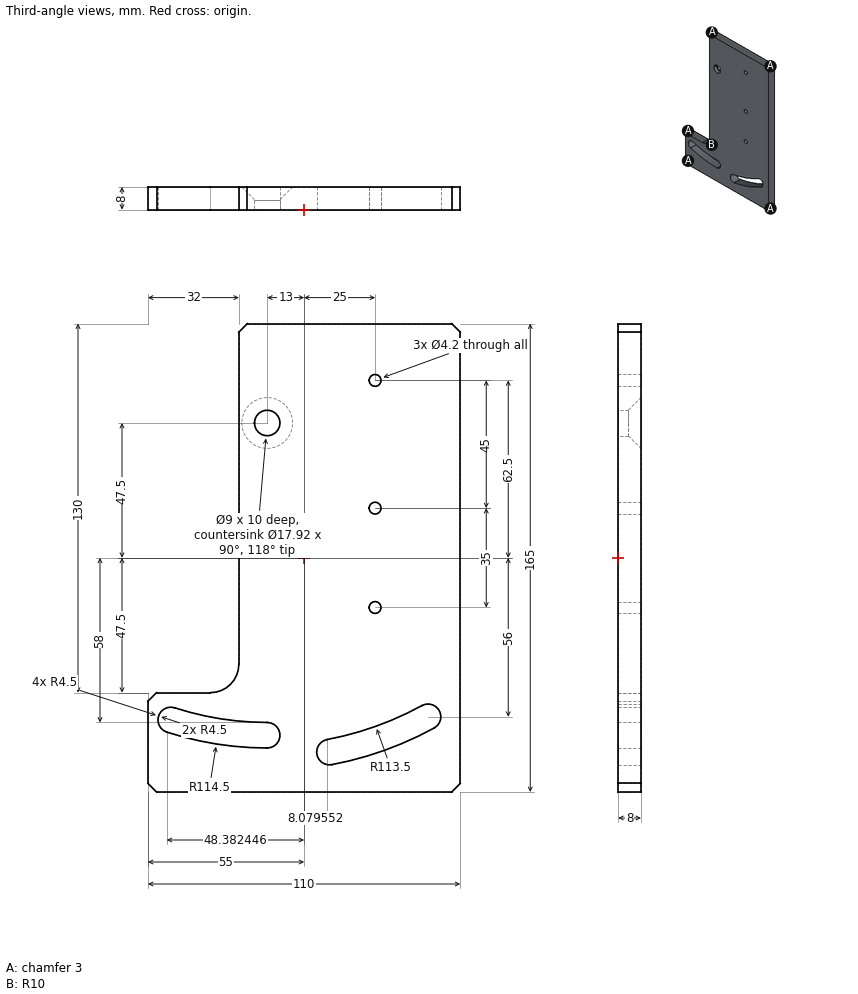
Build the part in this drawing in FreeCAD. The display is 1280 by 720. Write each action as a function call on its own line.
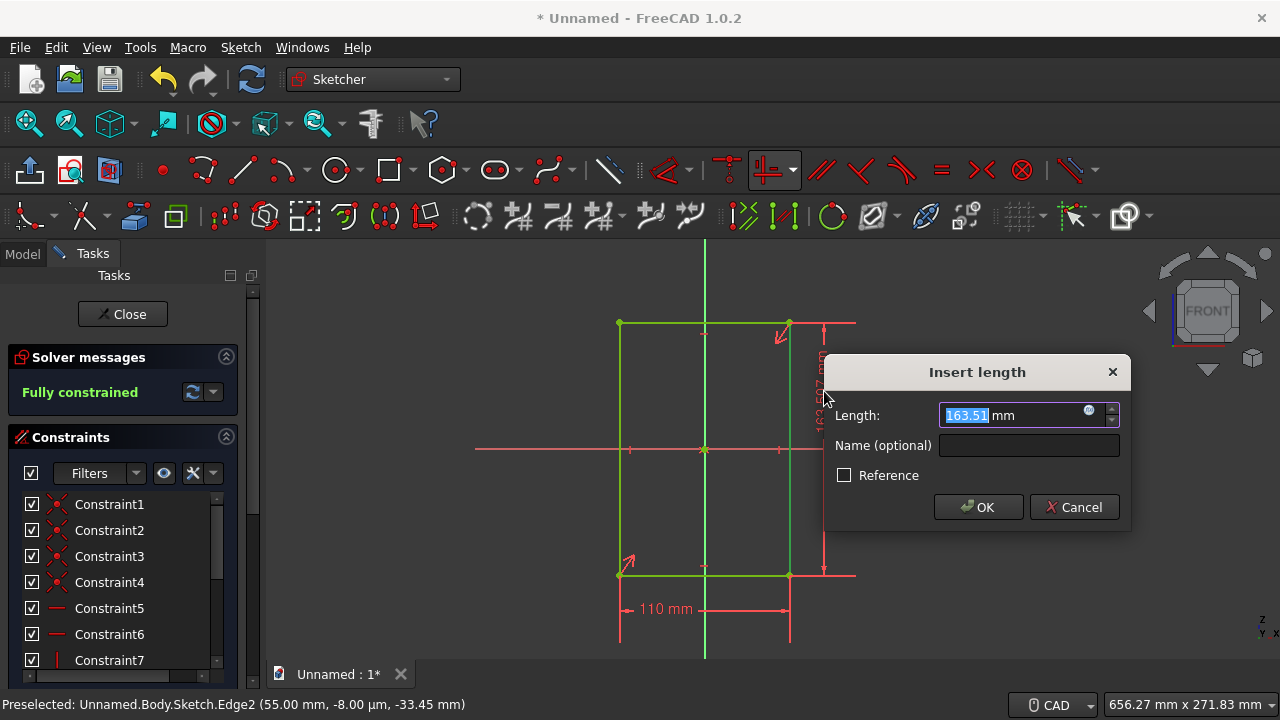
text(165)
key(Return)
key(Escape)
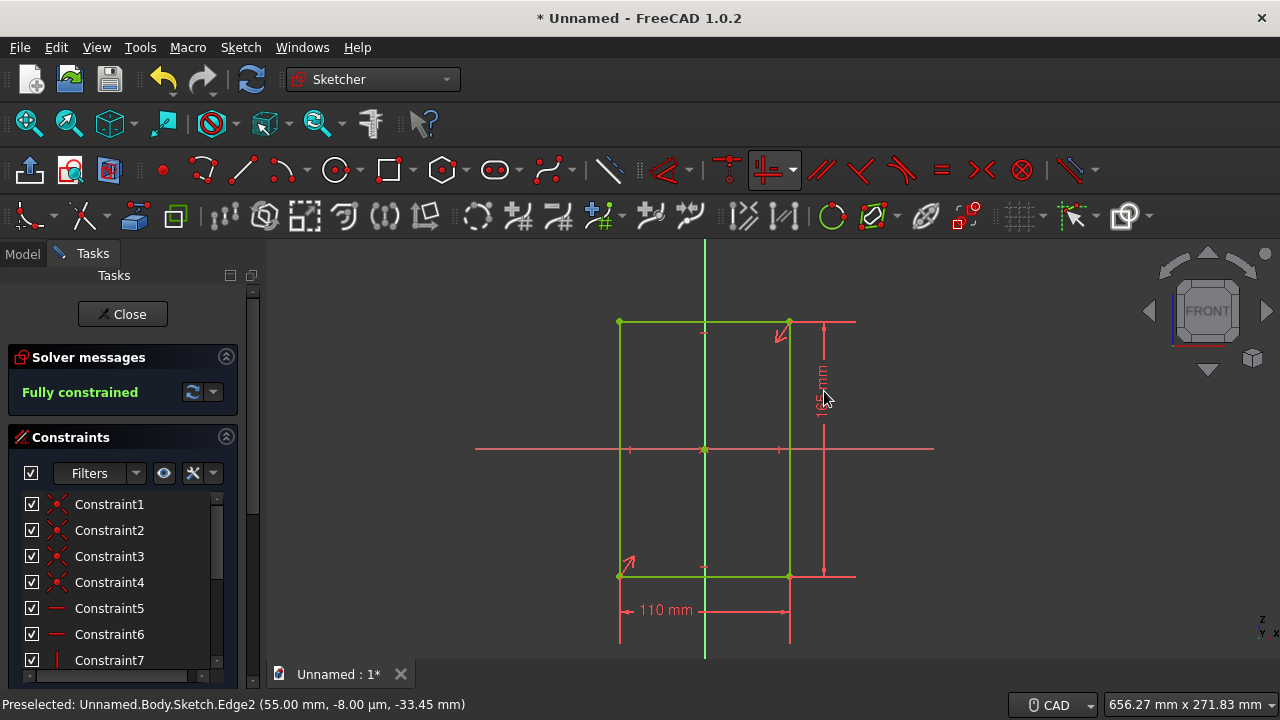
click(123, 314)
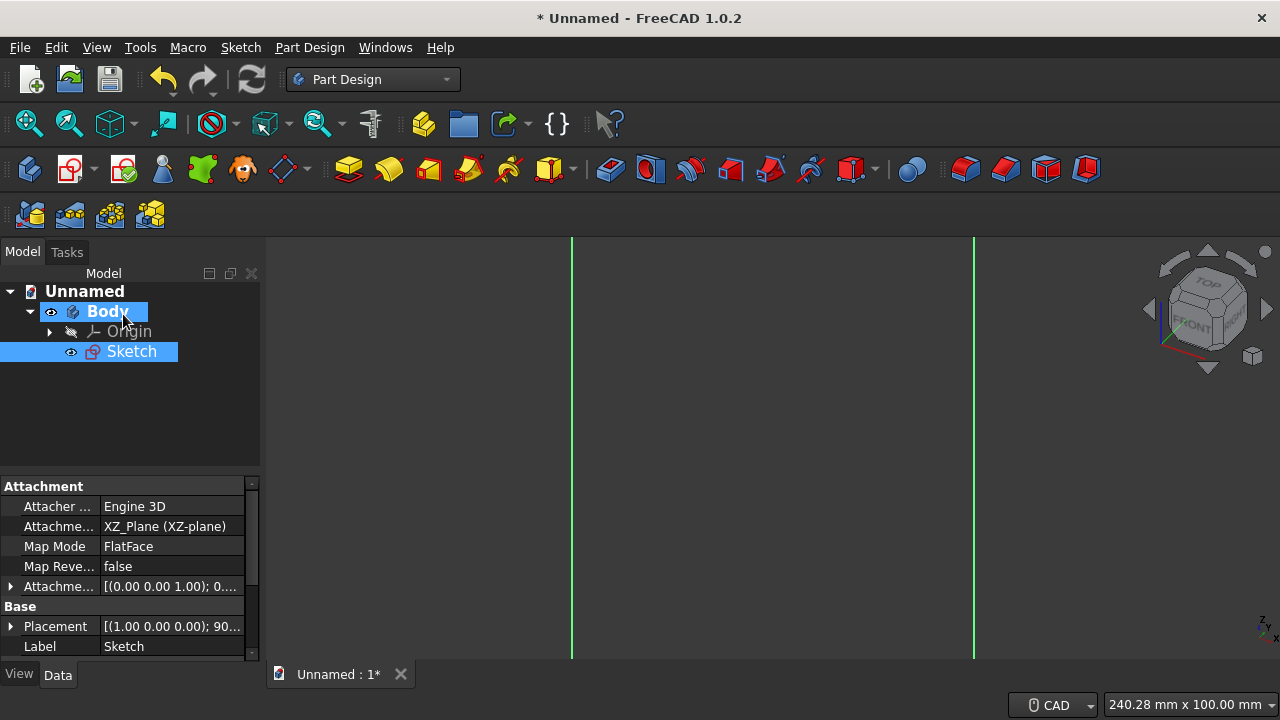
click(350, 170)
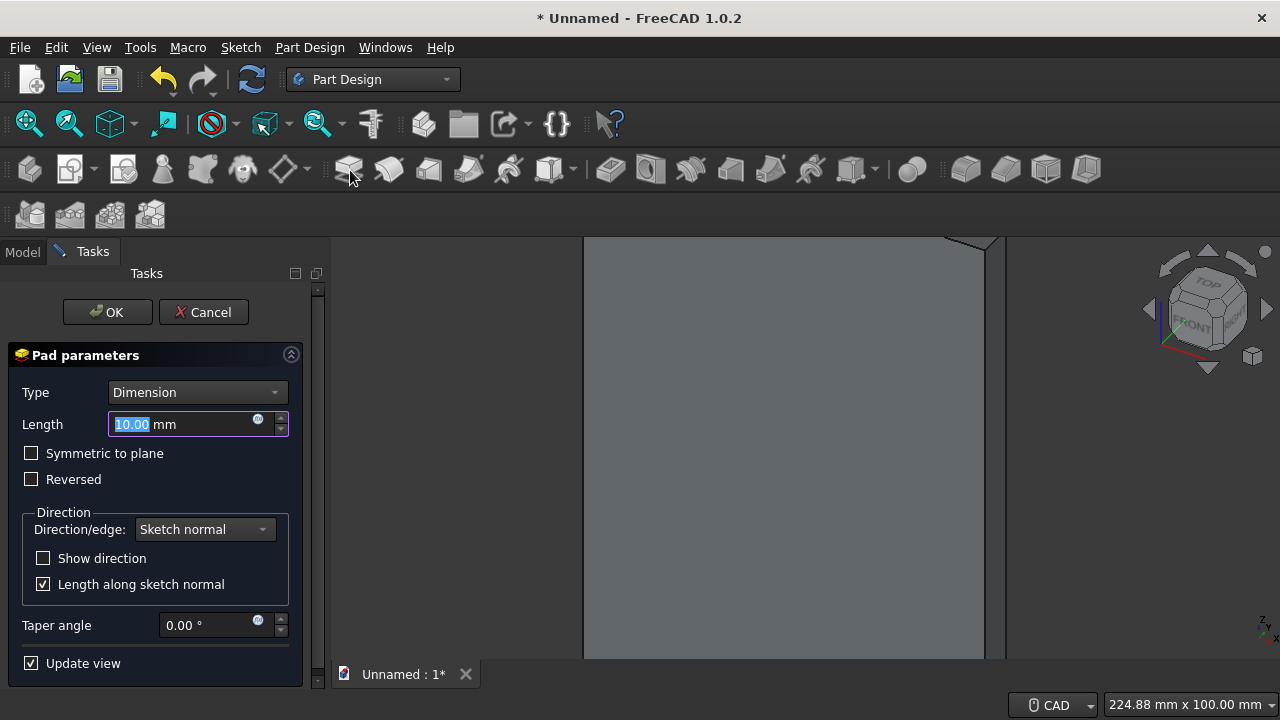
text(8)
key(Tab)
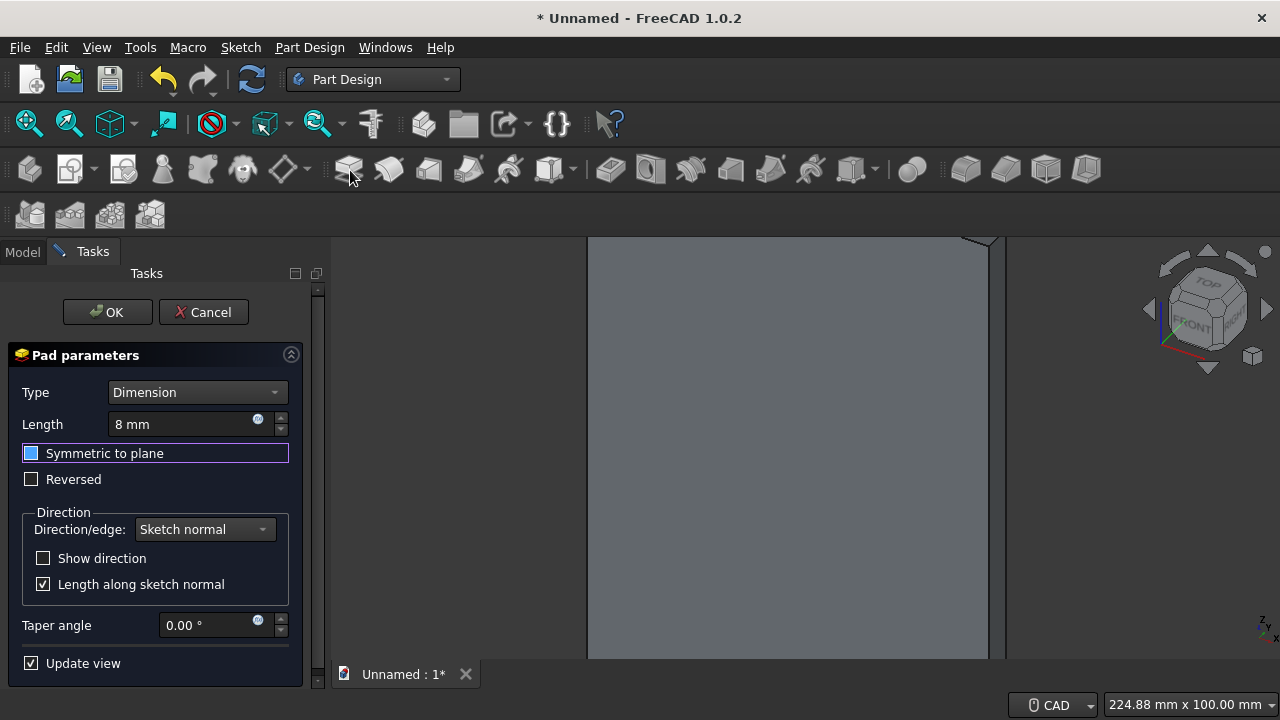
click(30, 479)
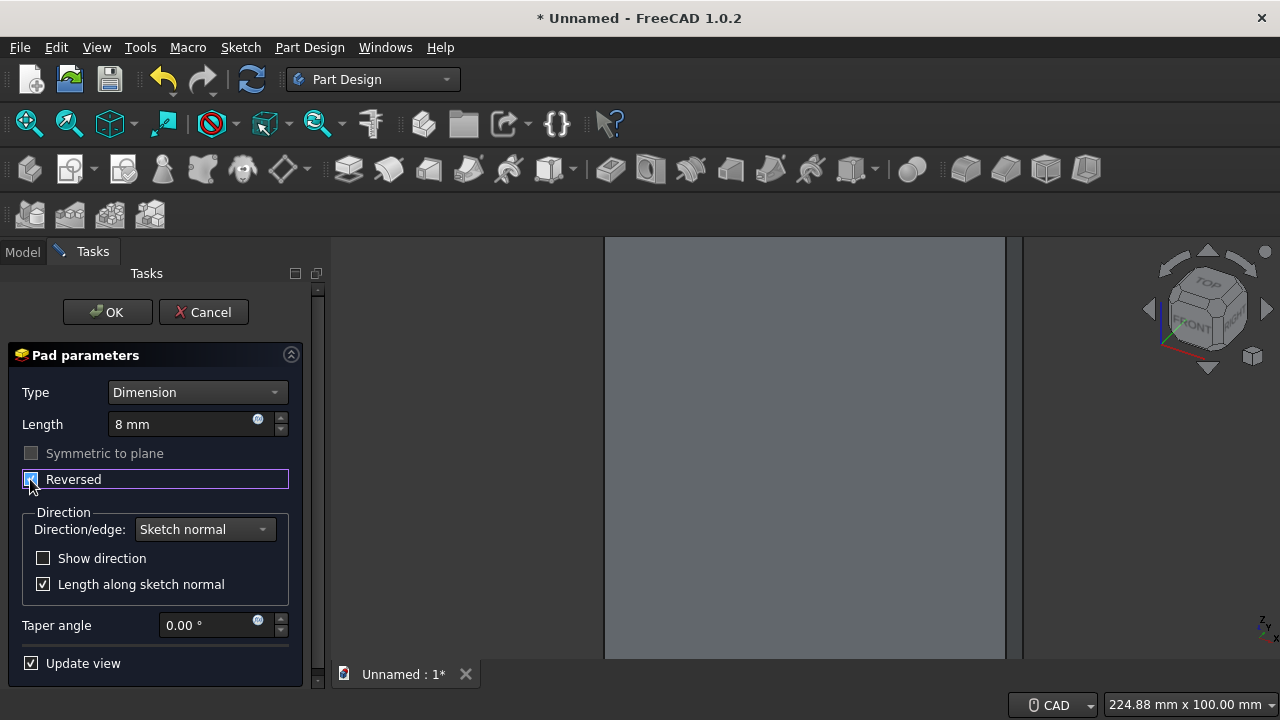
click(108, 312)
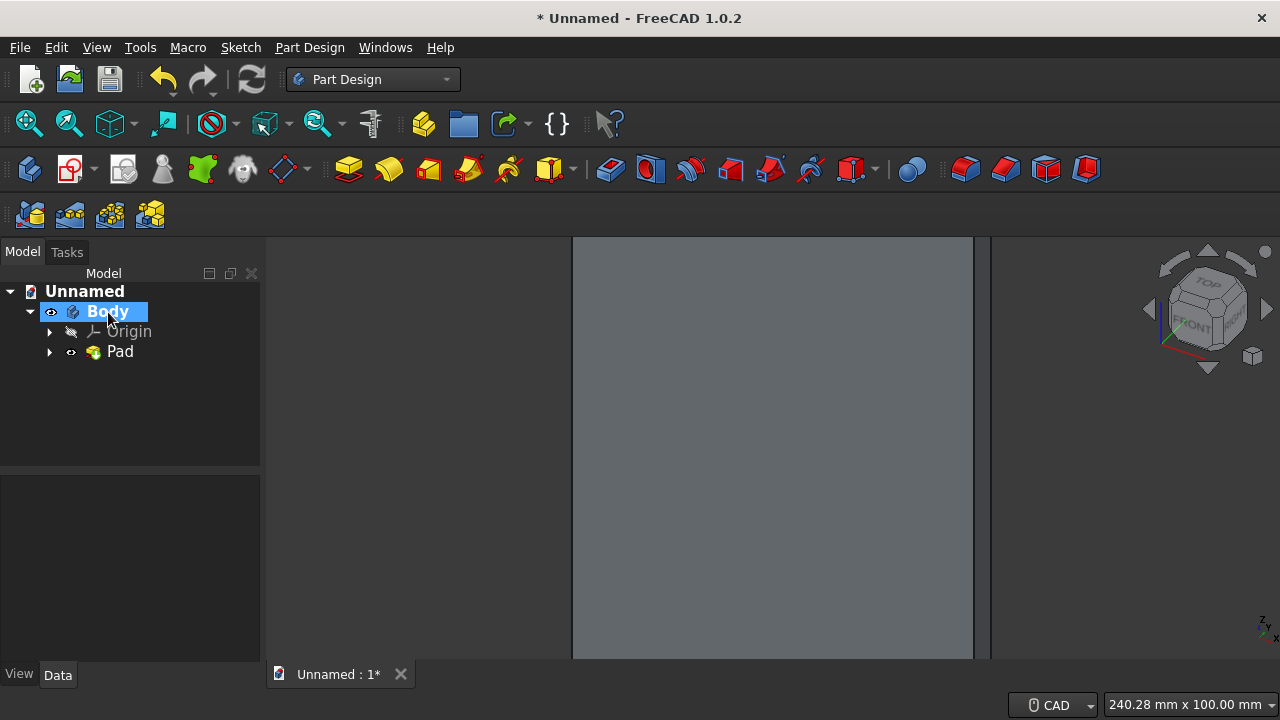
click(30, 124)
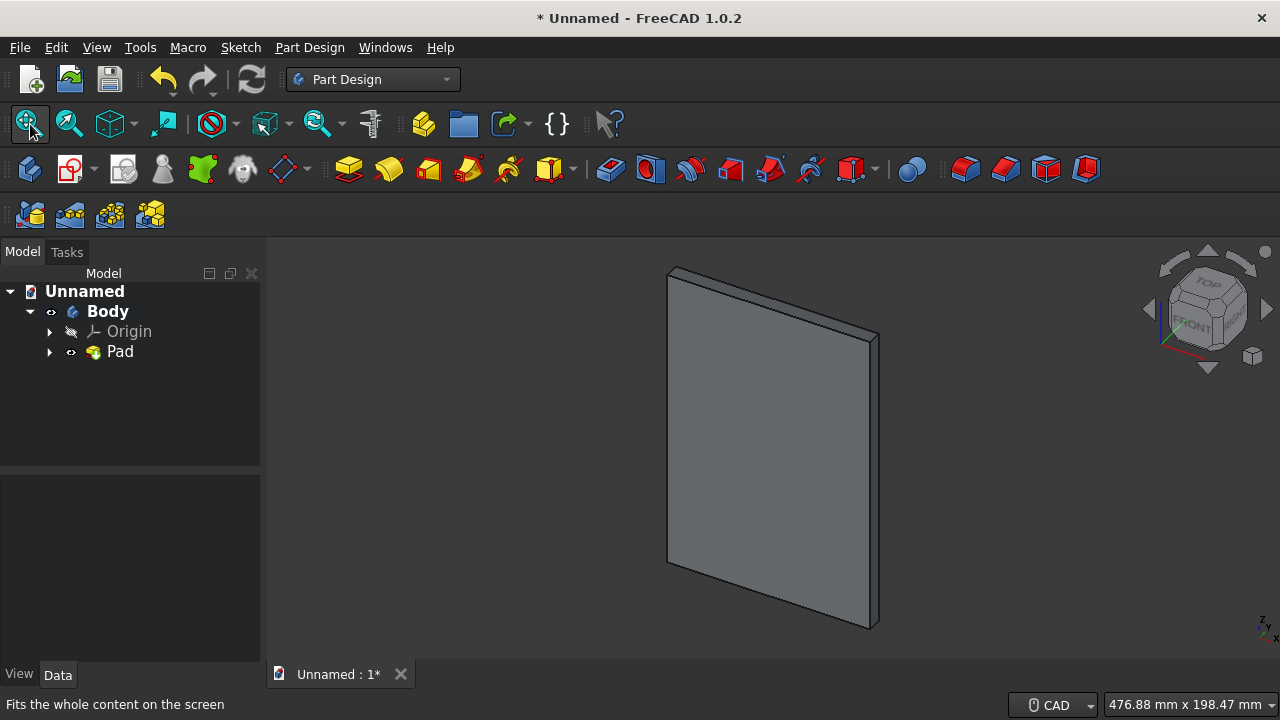
key(4)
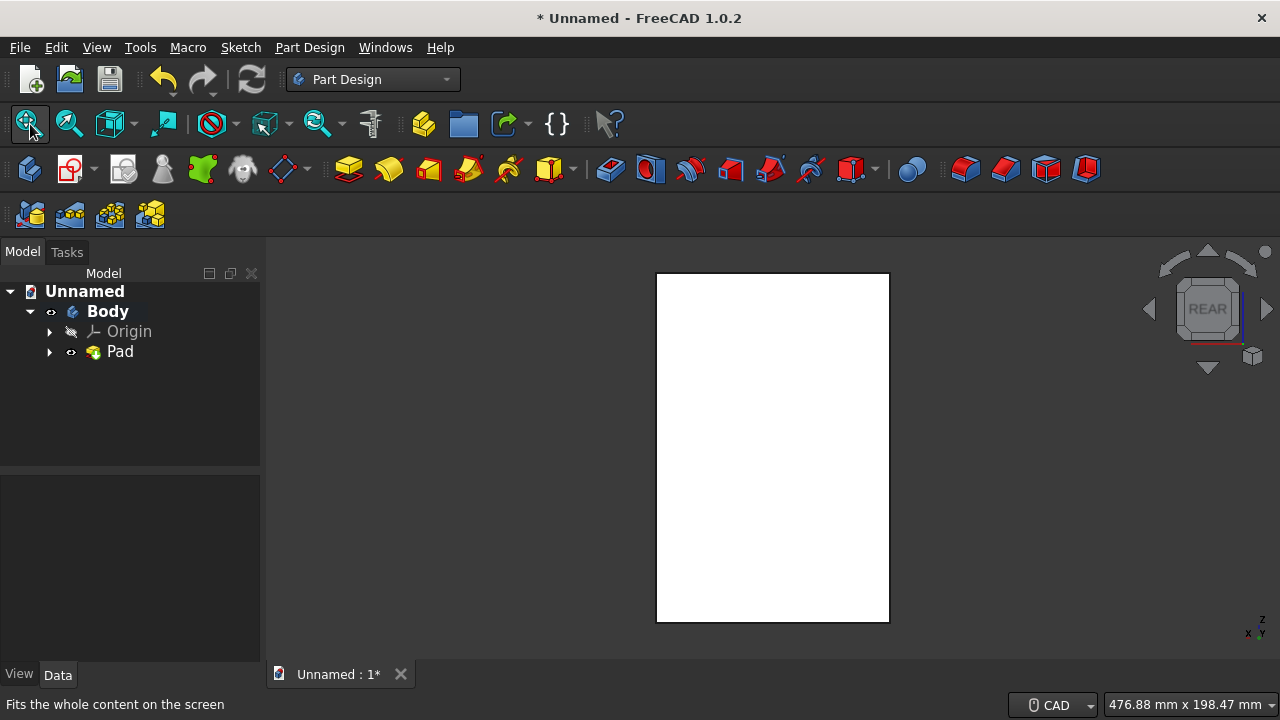
click(773, 397)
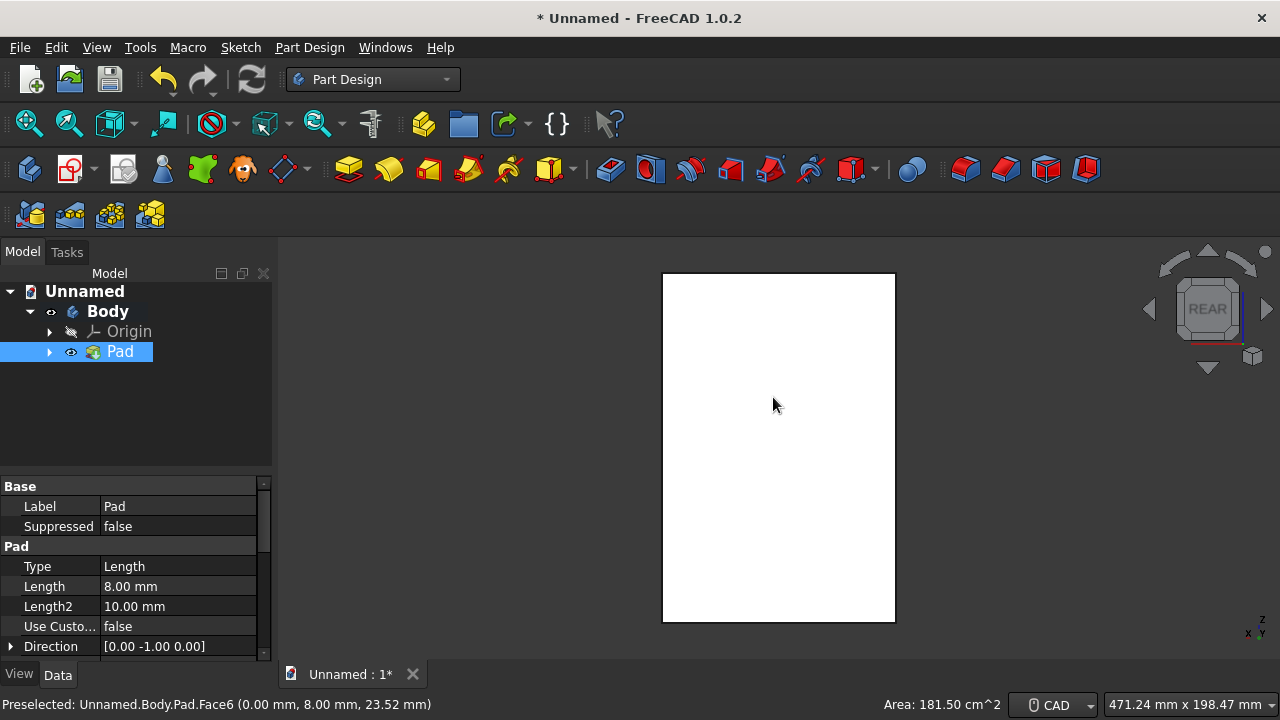
click(70, 170)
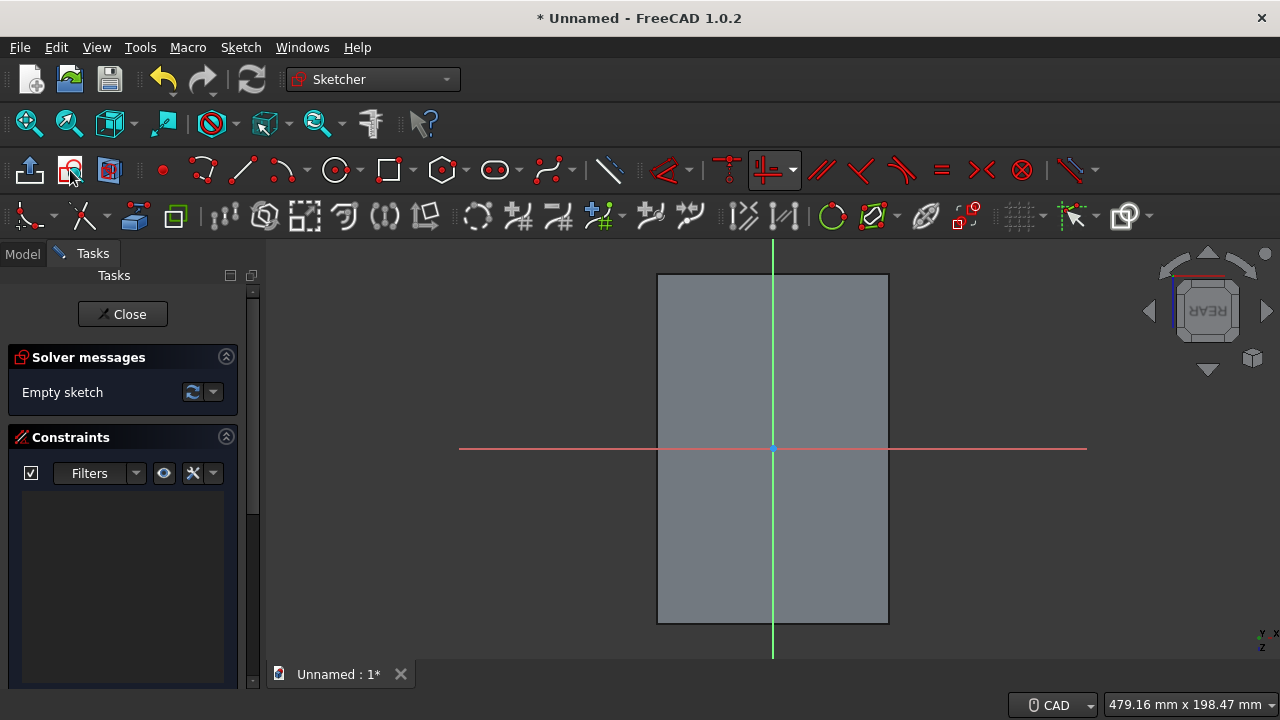
scroll(658, 282, down, 1)